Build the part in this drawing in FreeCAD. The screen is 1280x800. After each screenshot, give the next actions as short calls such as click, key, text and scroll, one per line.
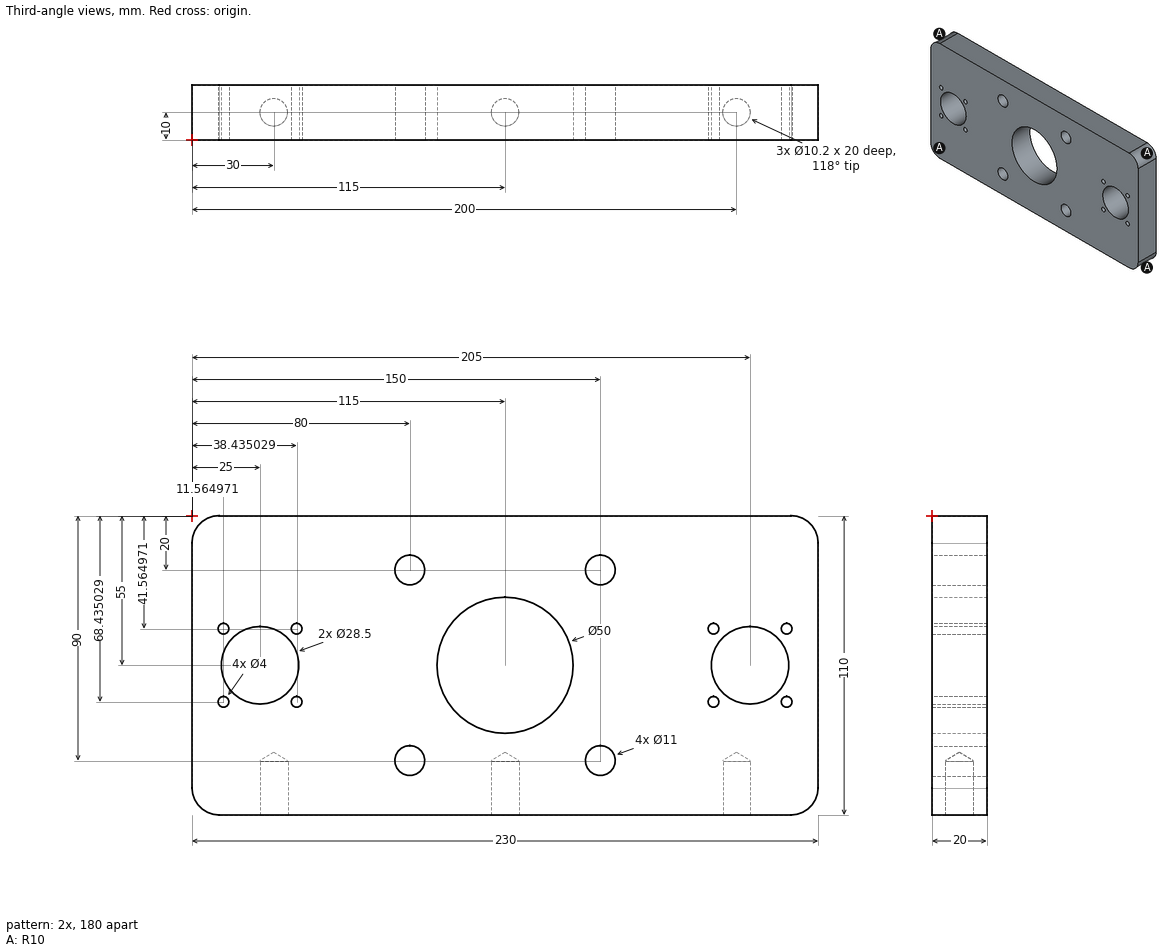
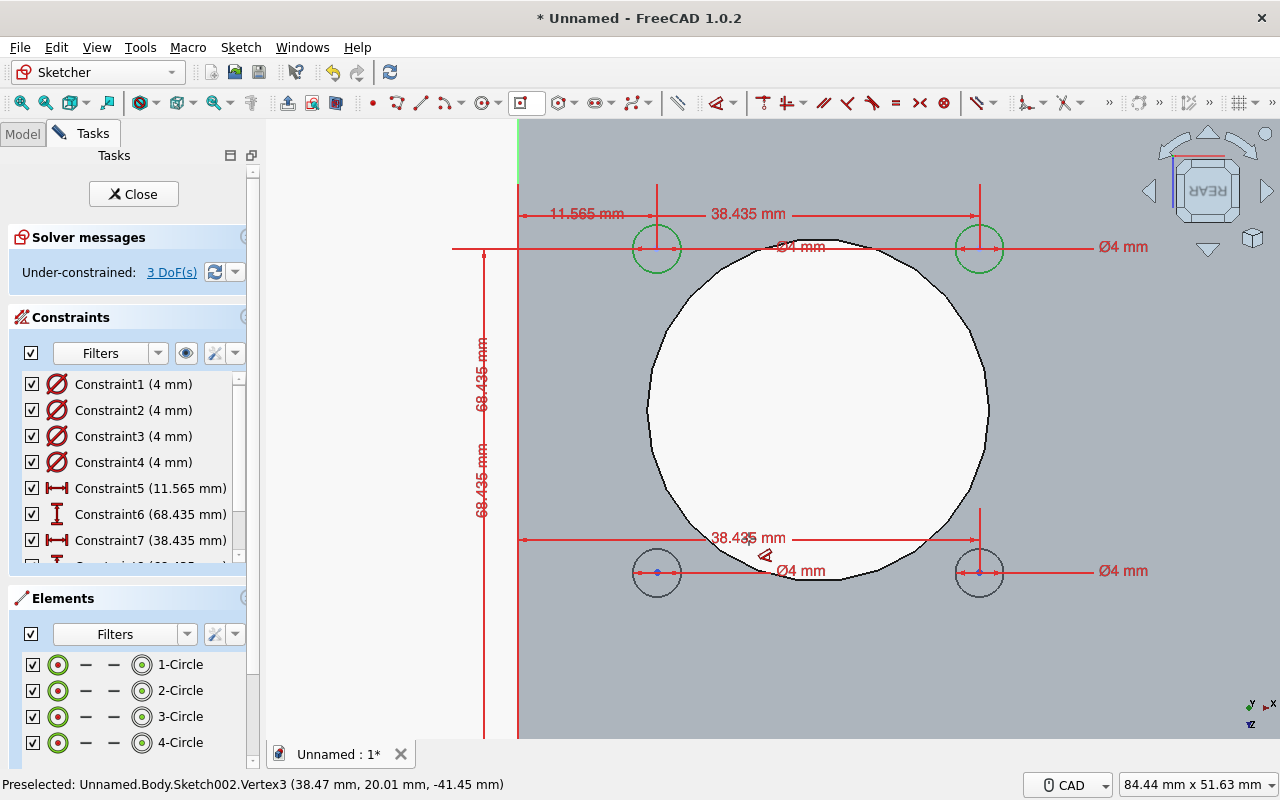
click(980, 573)
click(484, 642)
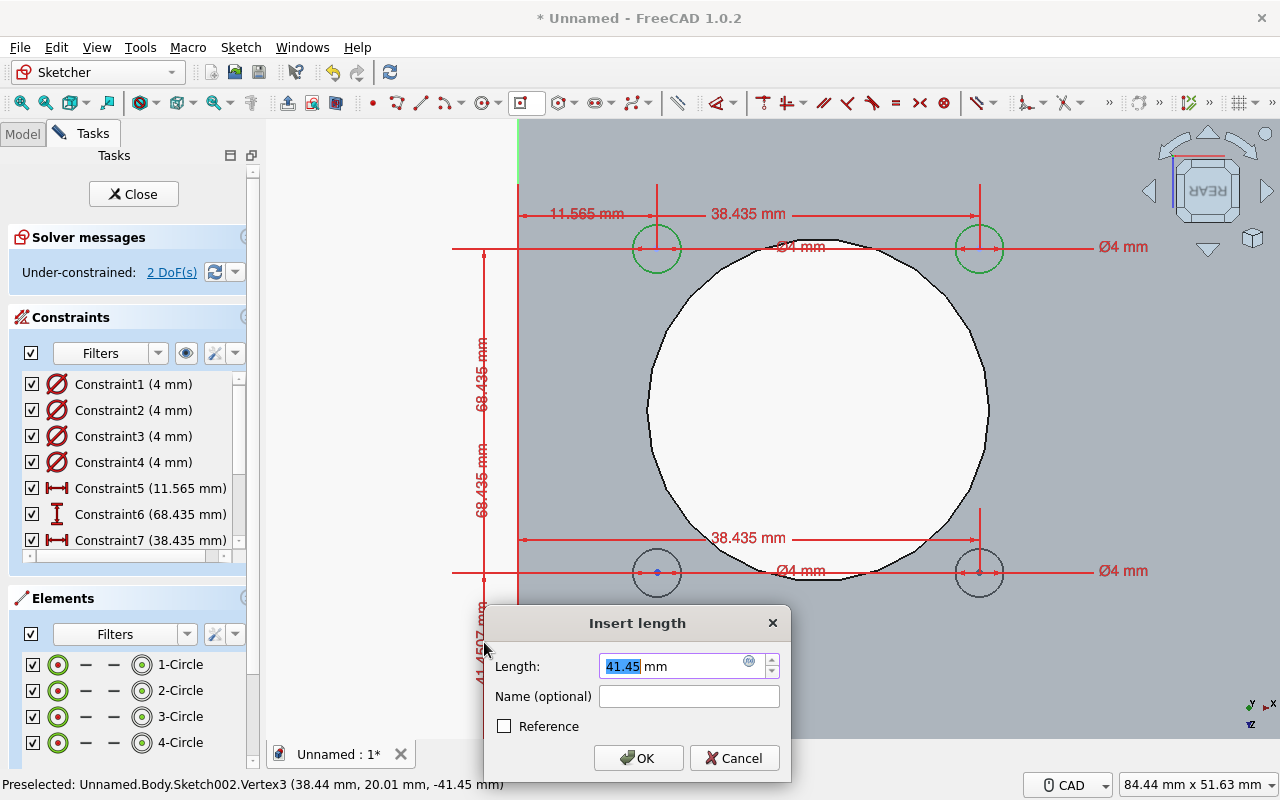
text(41.564971)
key(Return)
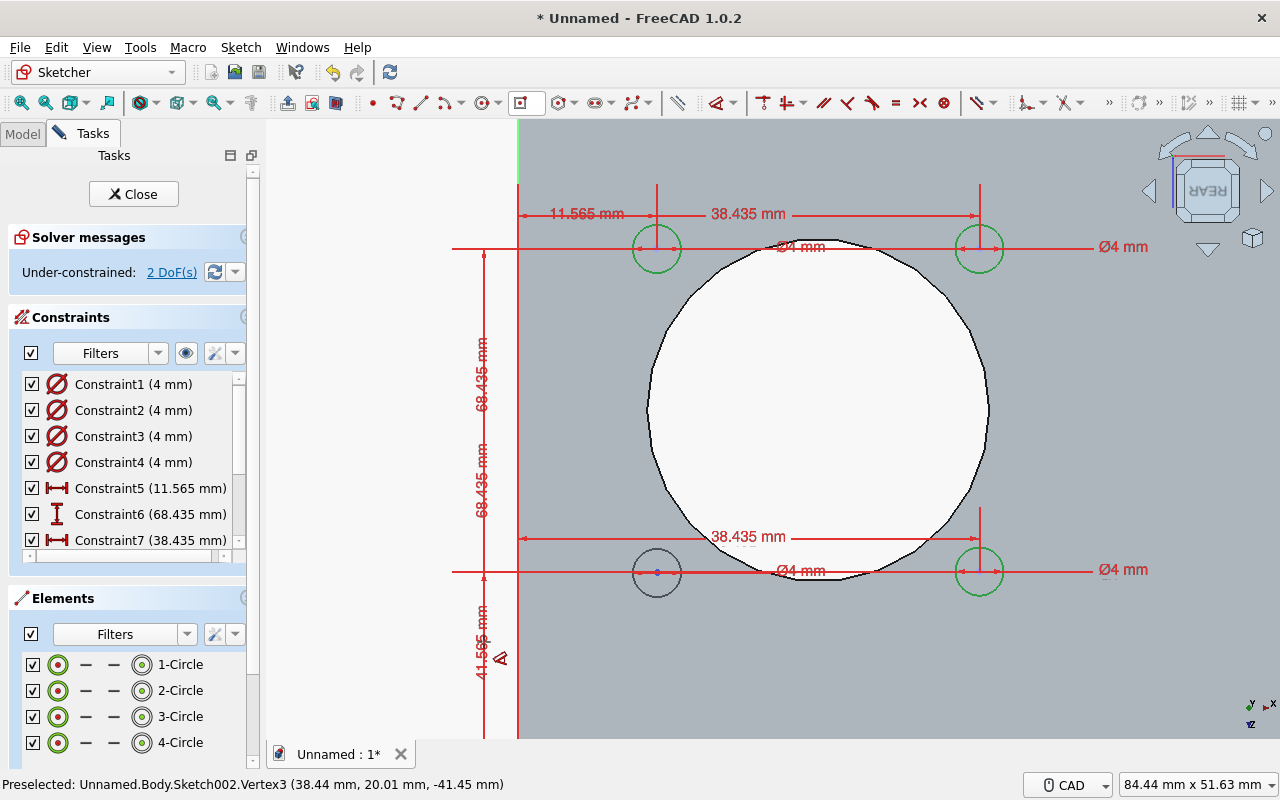
click(657, 573)
click(587, 539)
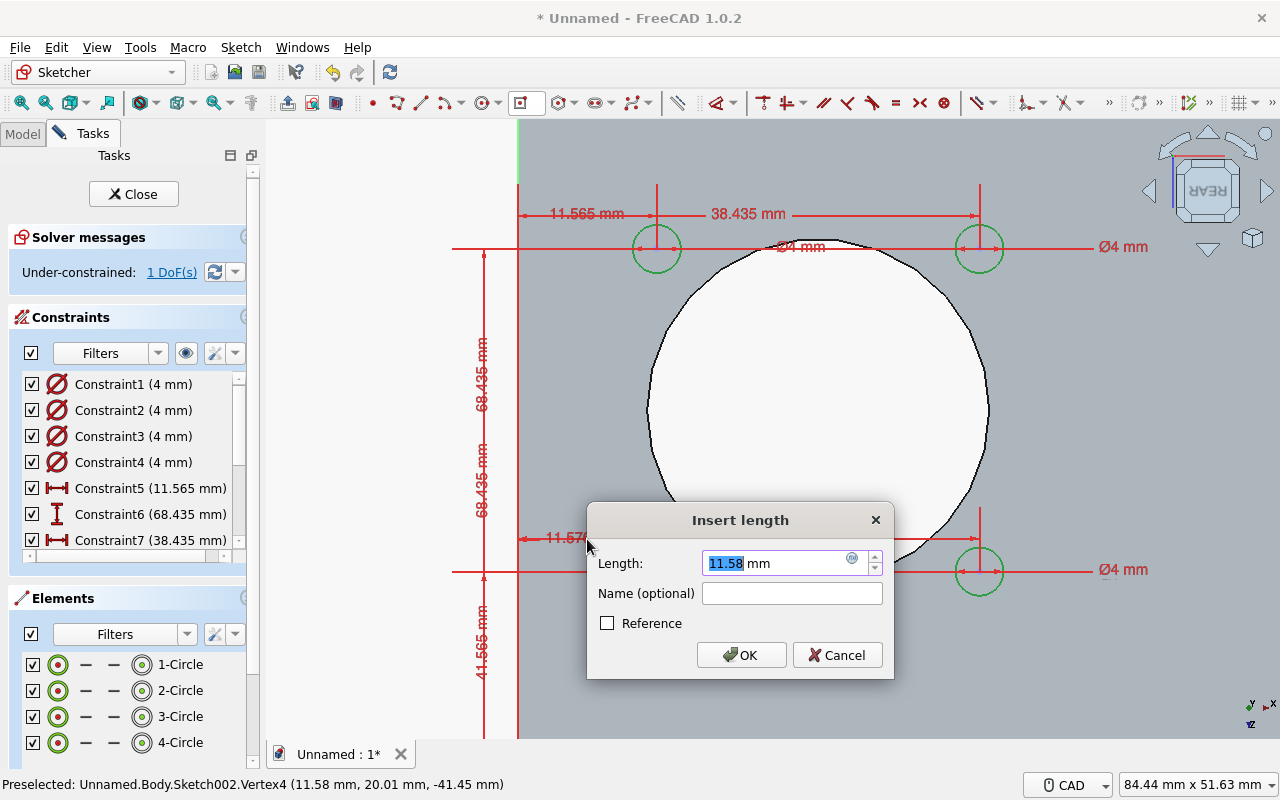
text(11.564971)
key(Return)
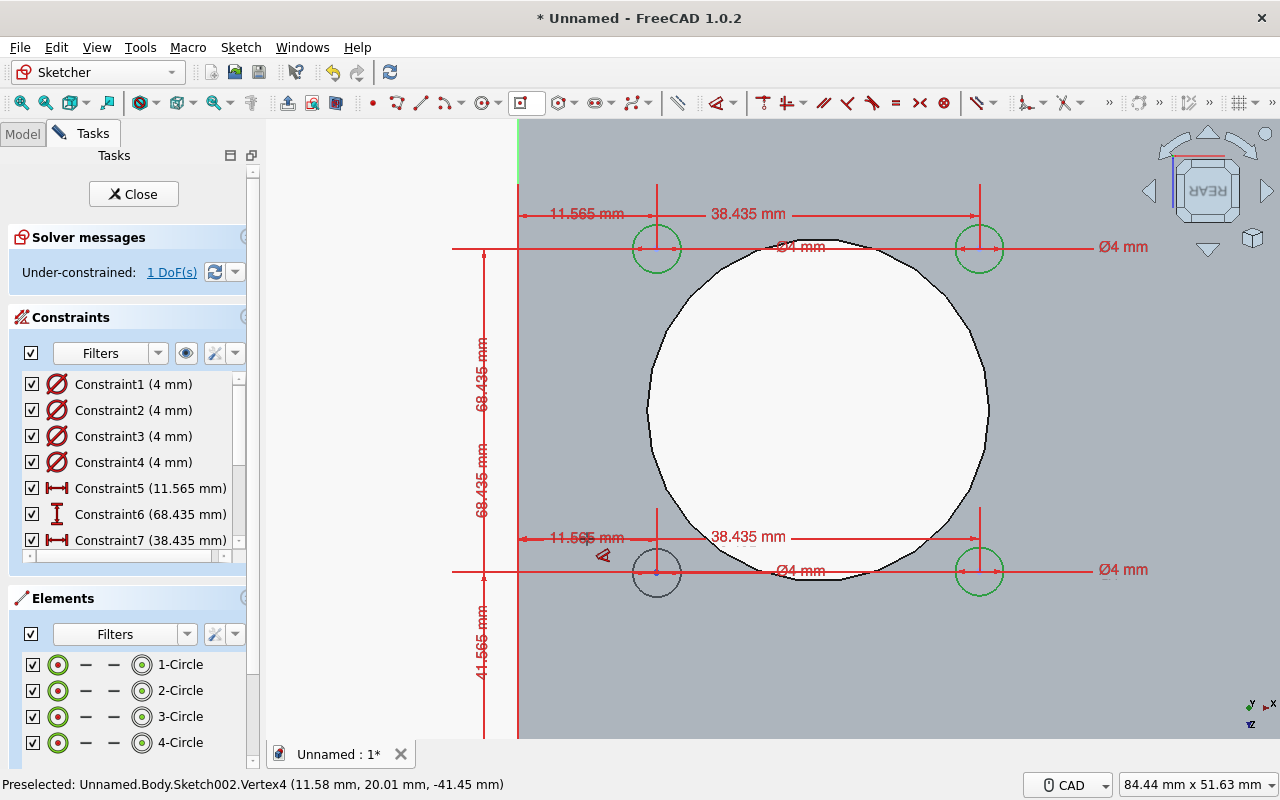
click(657, 573)
click(484, 610)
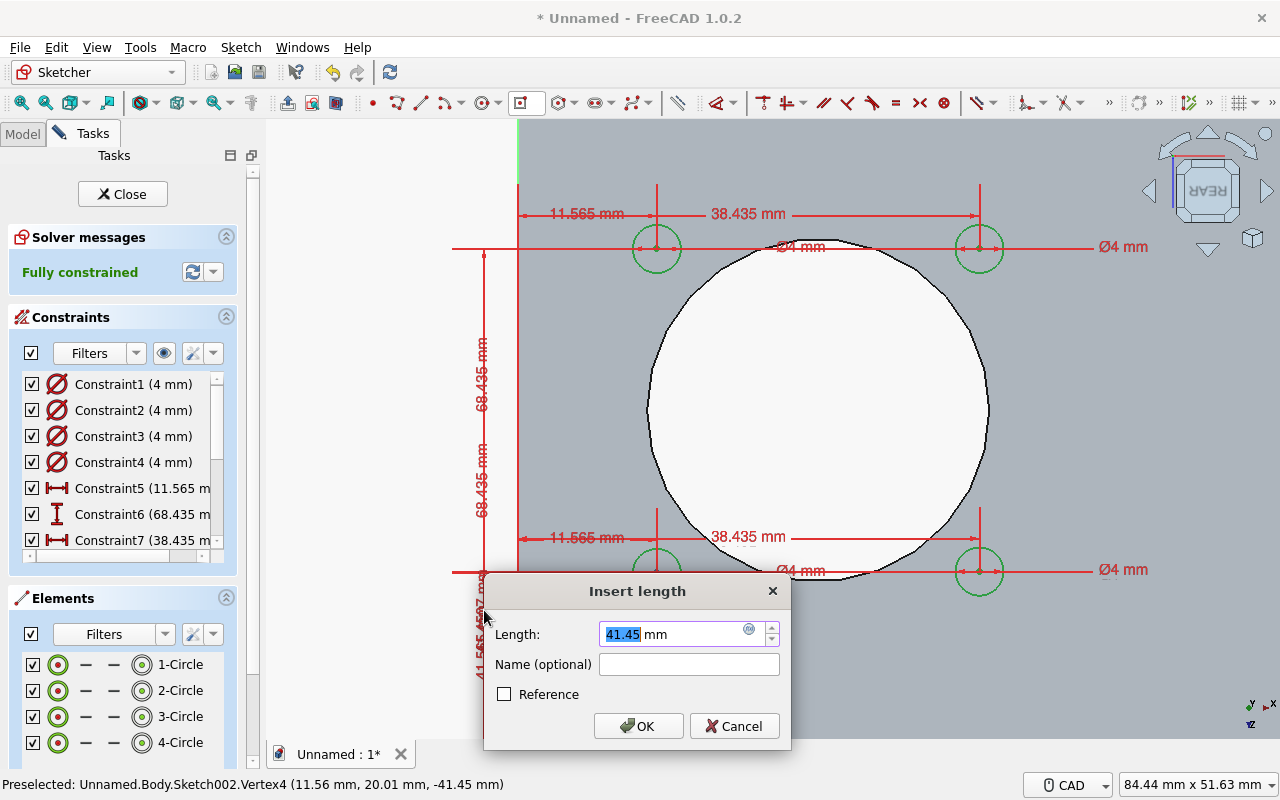
text(41.564971)
key(Return)
key(Escape)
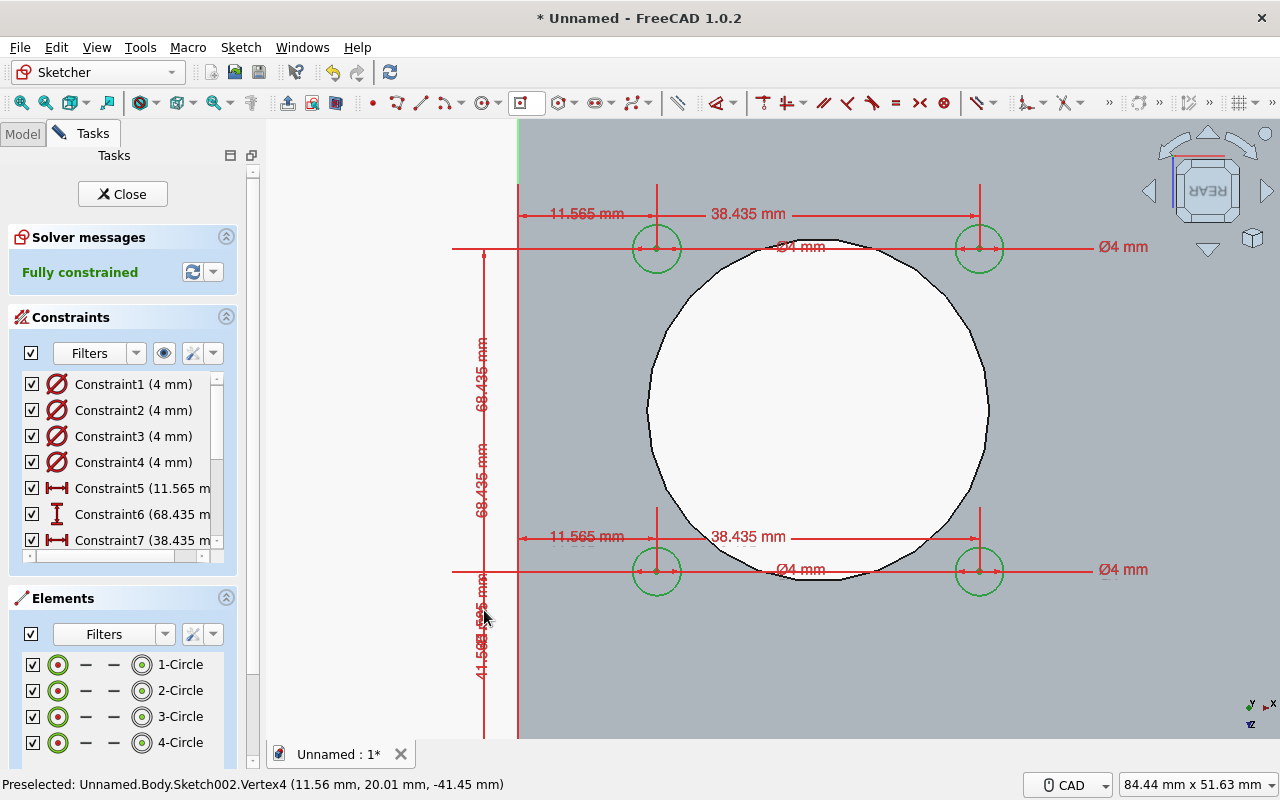
click(123, 194)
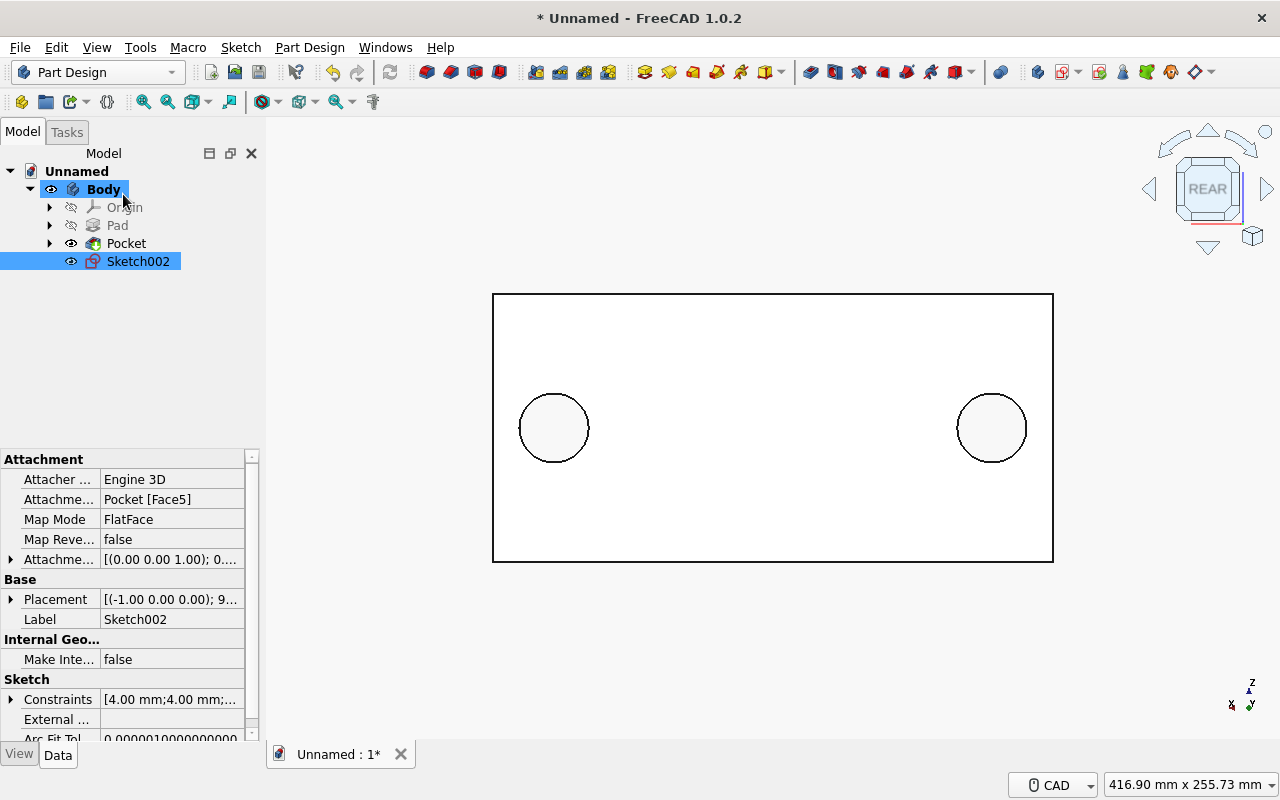
click(812, 72)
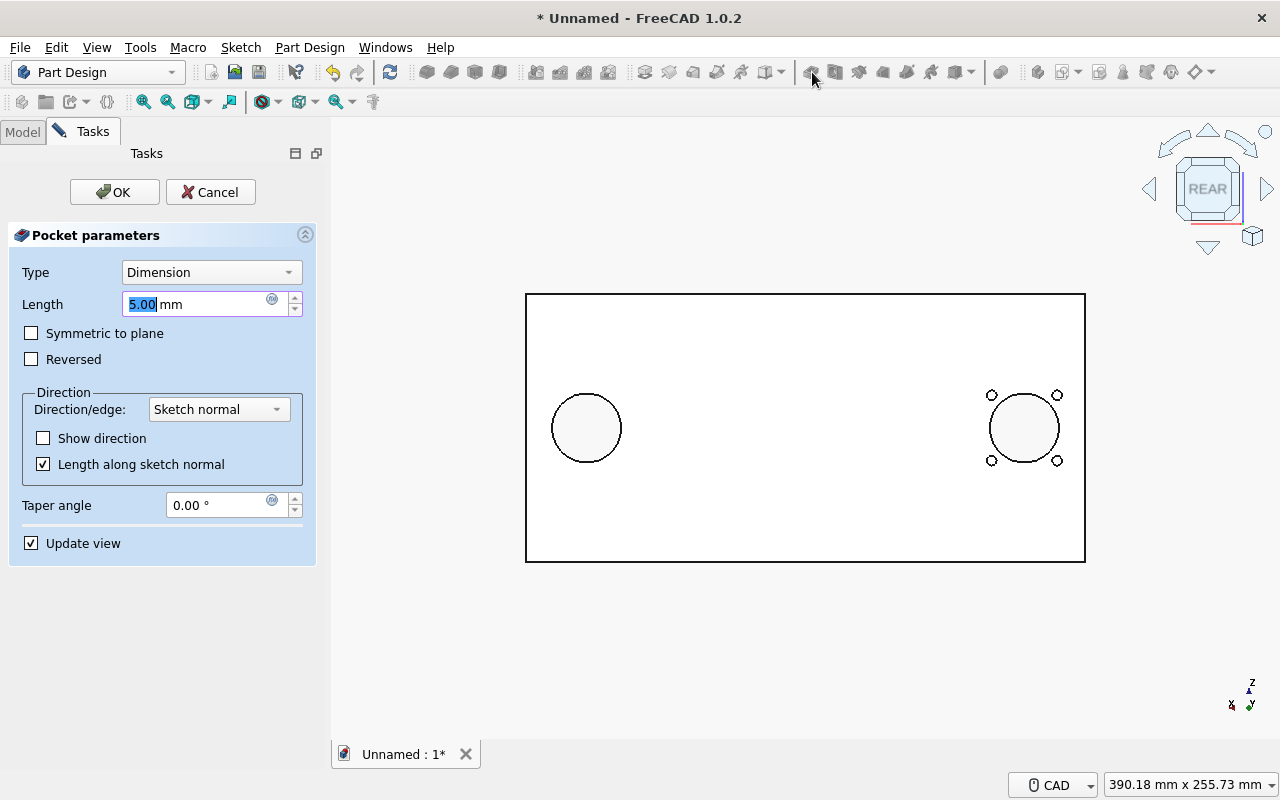
click(212, 272)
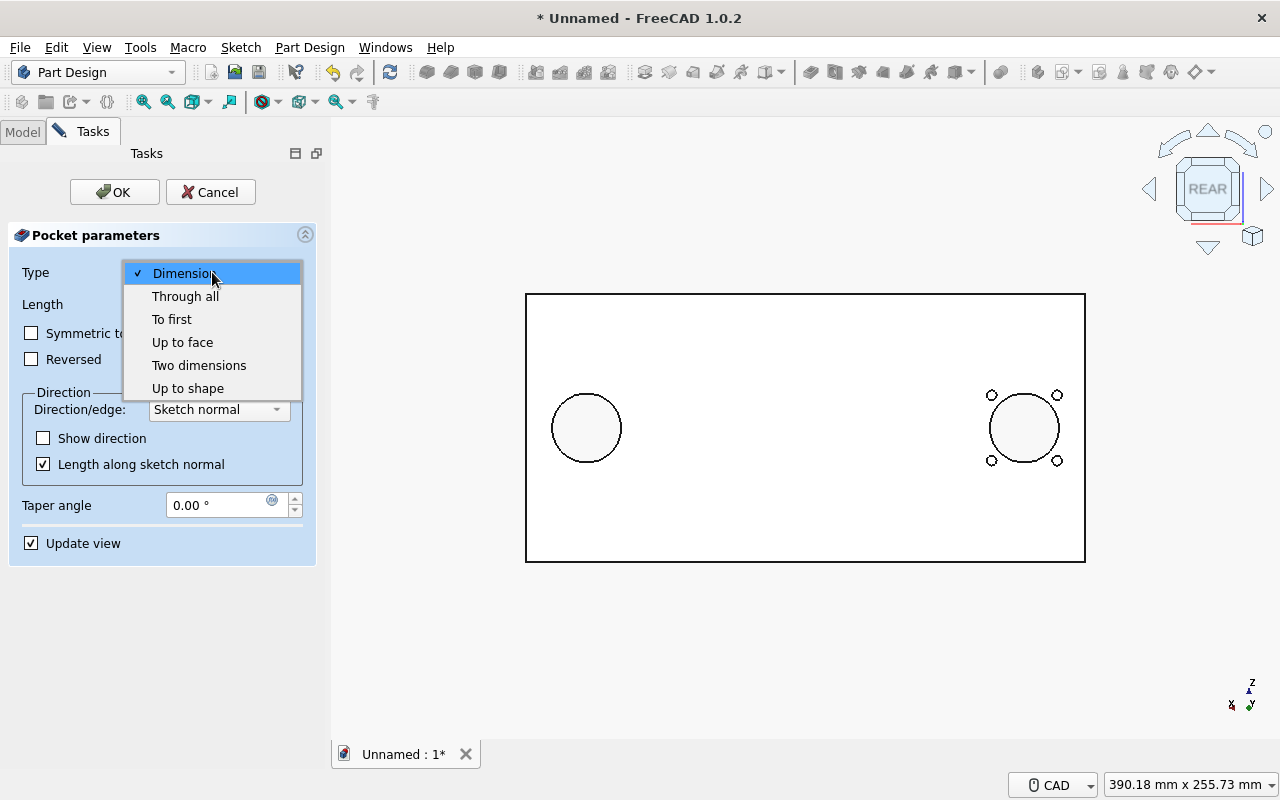
click(212, 296)